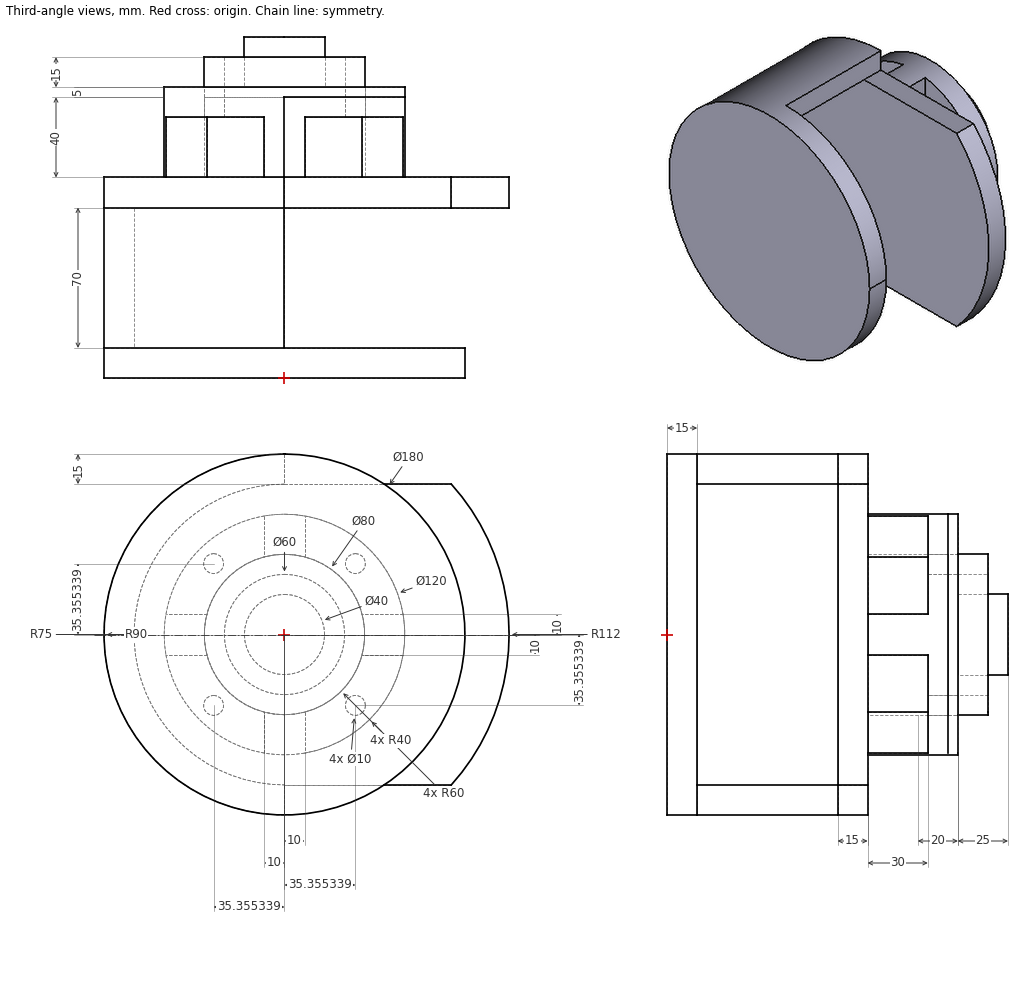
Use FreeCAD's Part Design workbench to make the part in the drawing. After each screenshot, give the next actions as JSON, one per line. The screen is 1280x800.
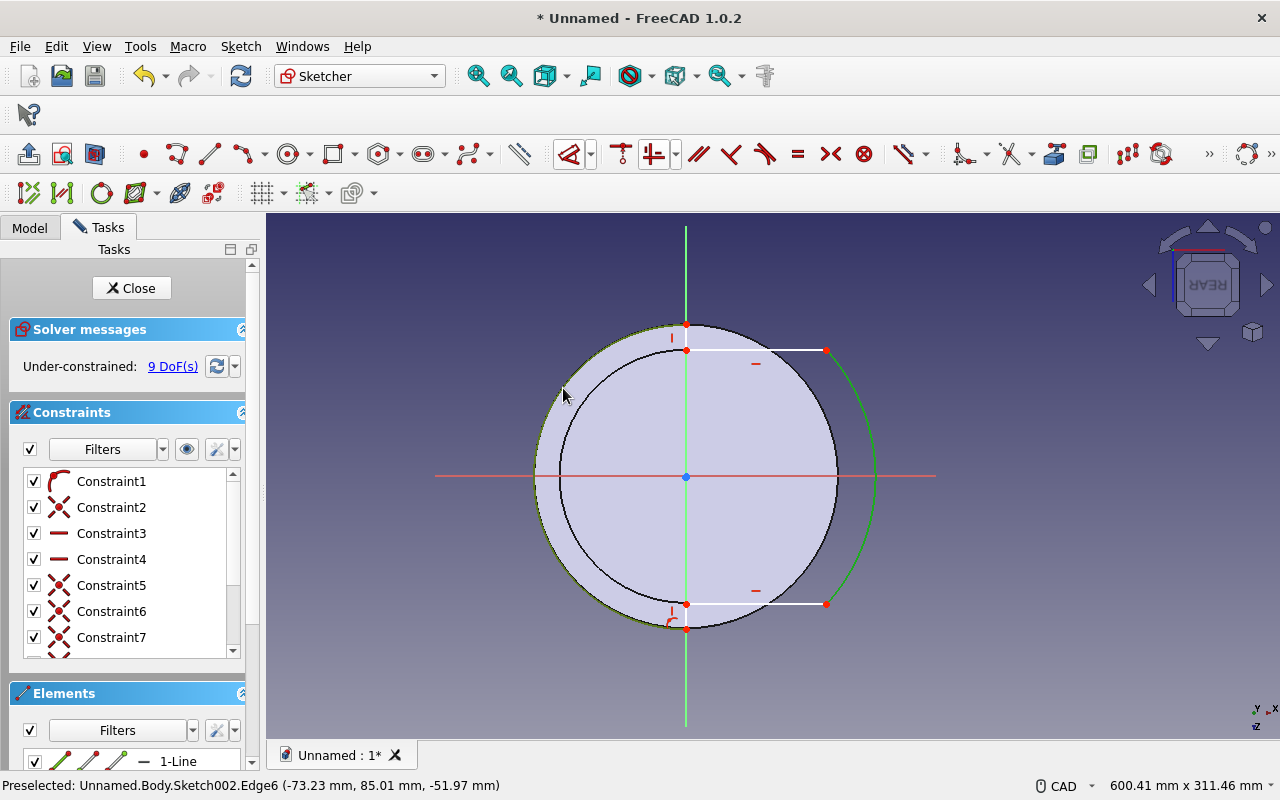
{"action": "left_click", "coordinate": [621, 154]}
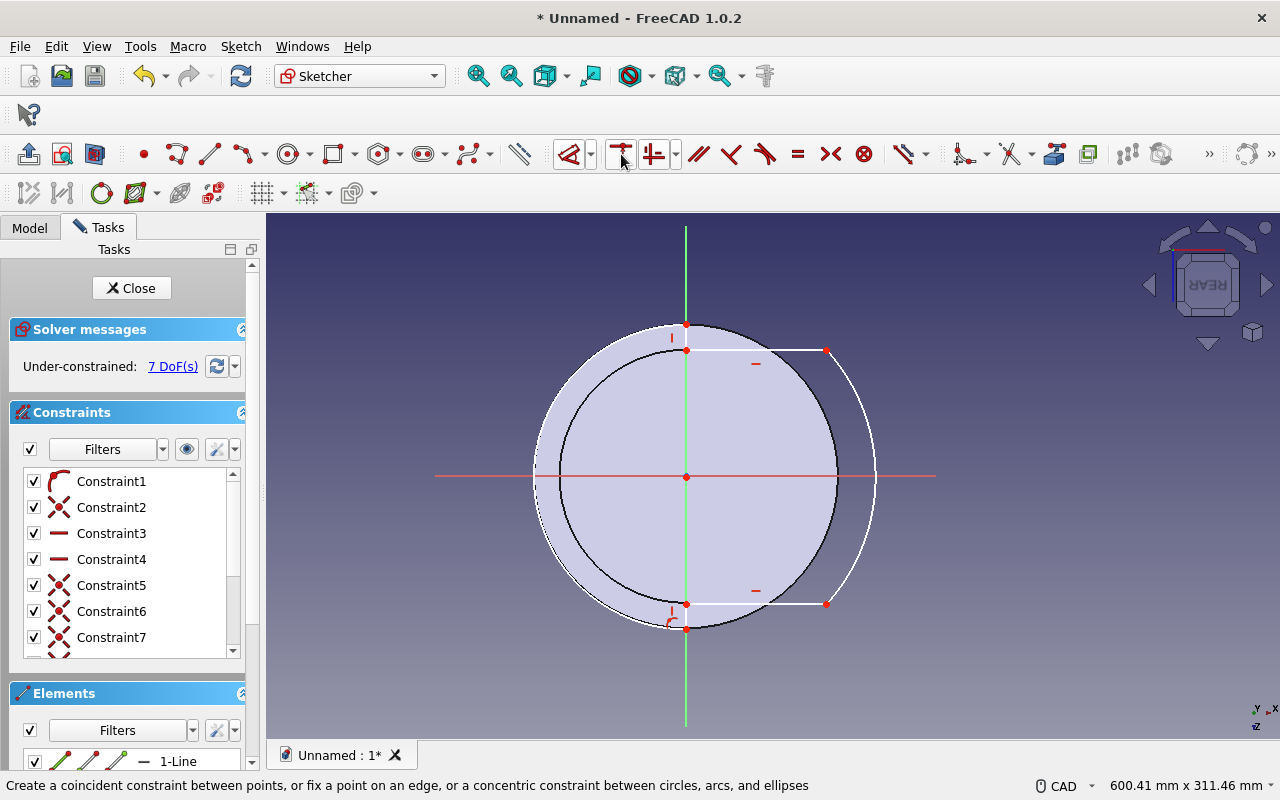
{"action": "left_click_drag", "start_coordinate": [676, 466], "coordinate": [696, 487]}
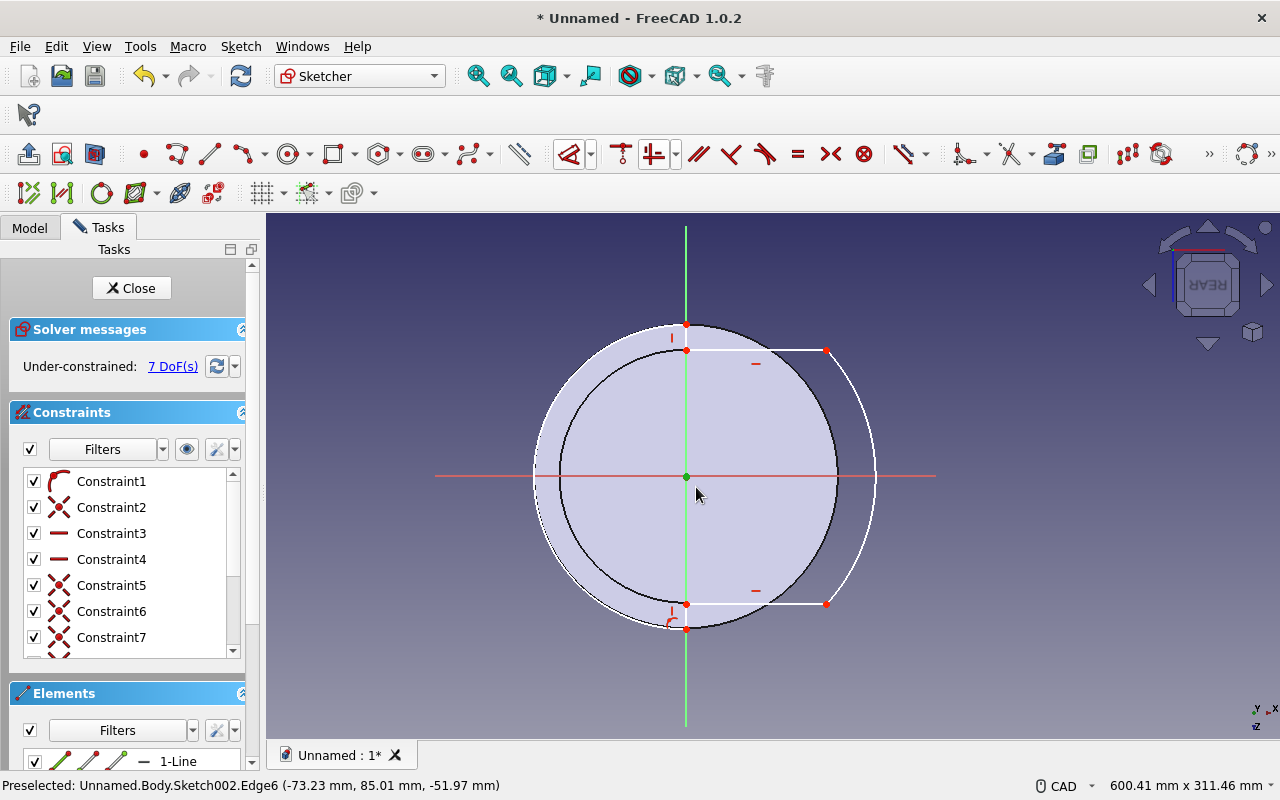
{"action": "left_click", "coordinate": [621, 154]}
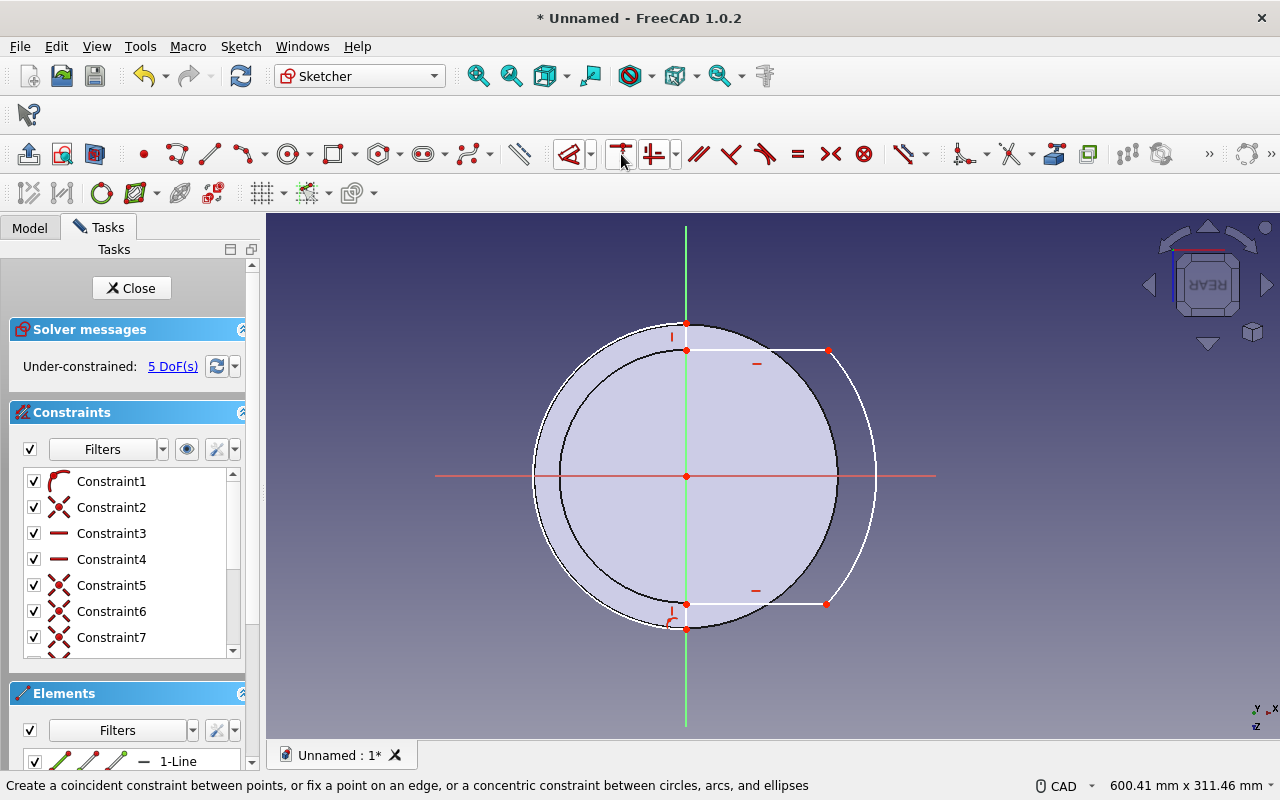
{"action": "left_click", "coordinate": [686, 604]}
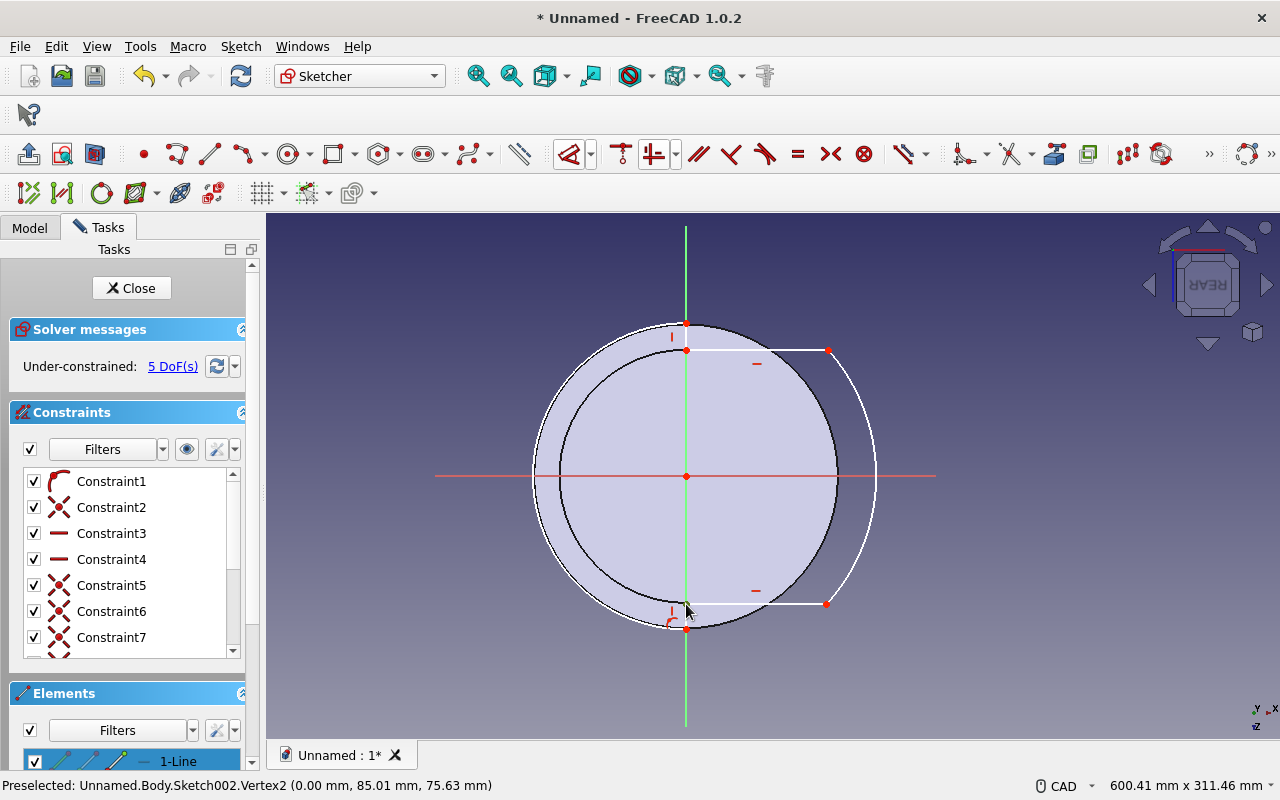
{"action": "left_click", "coordinate": [686, 350]}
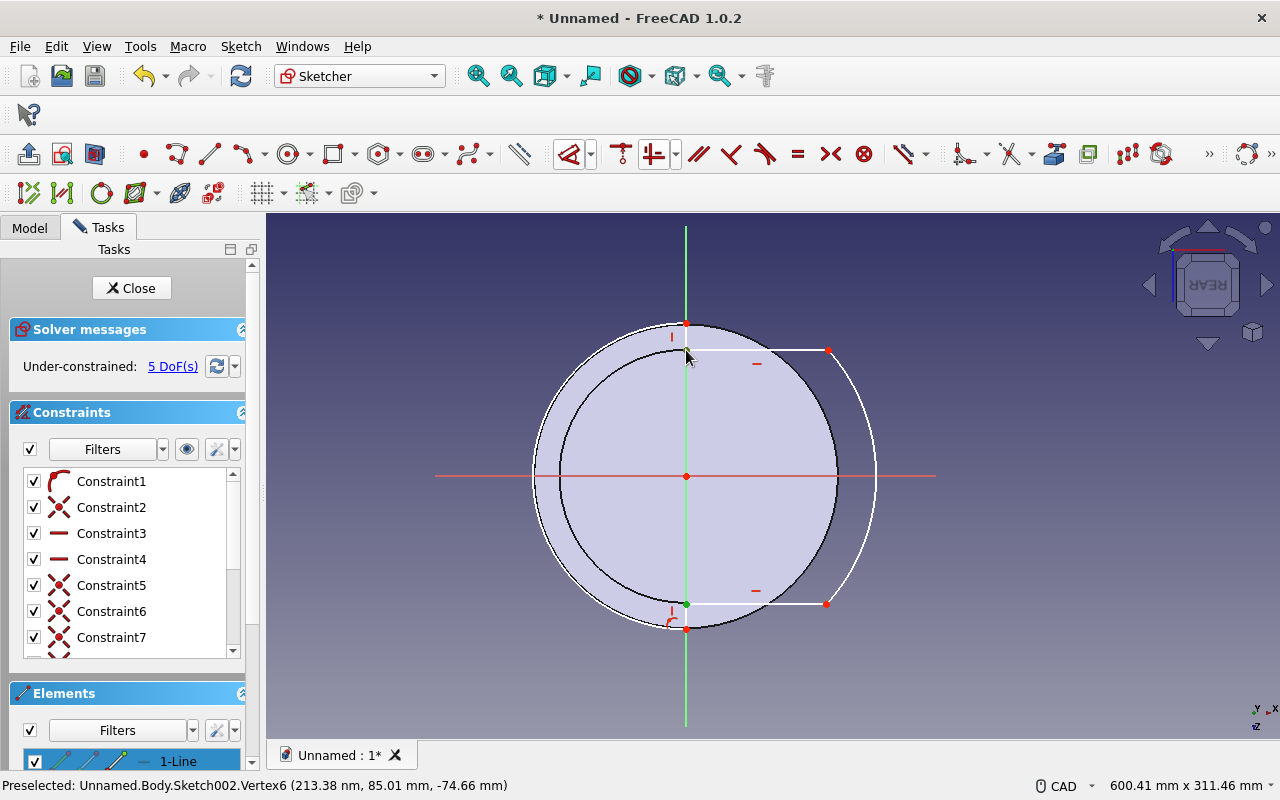
{"action": "left_click", "coordinate": [470, 476]}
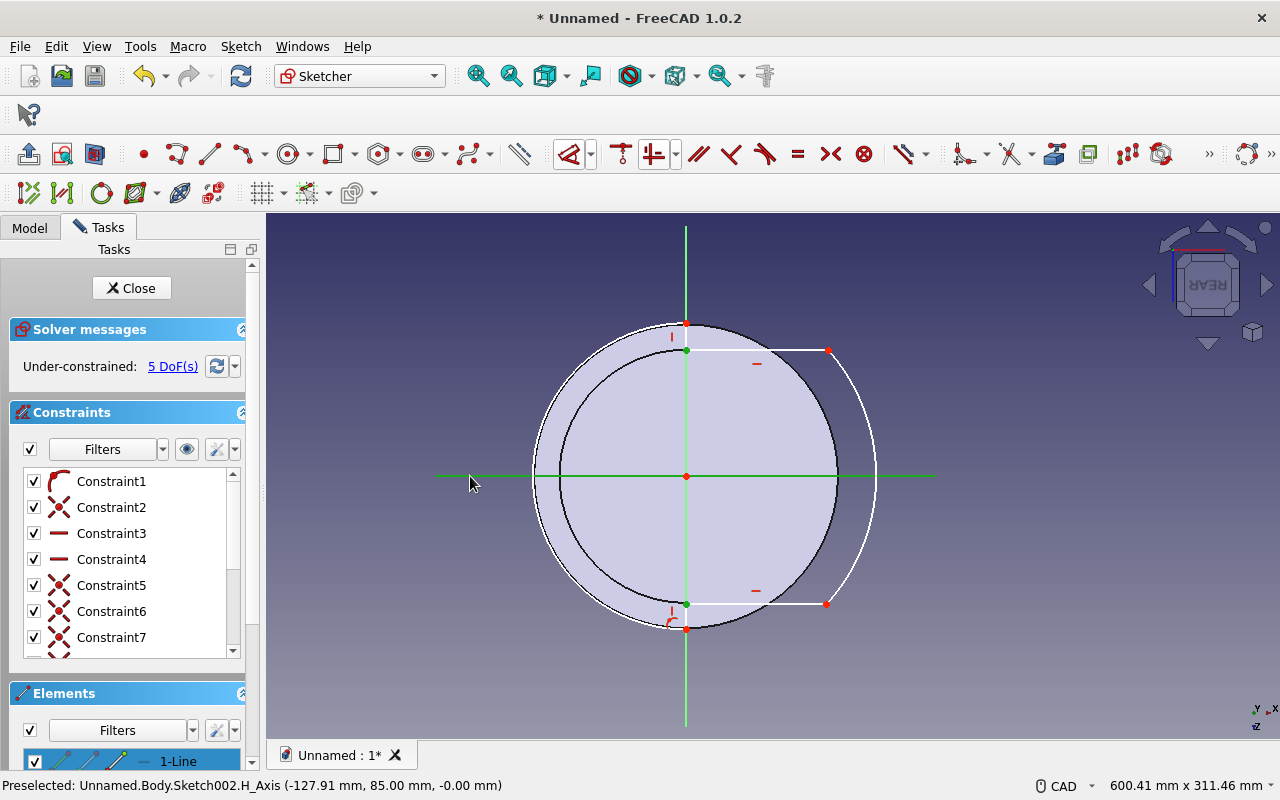
{"action": "left_click", "coordinate": [831, 154]}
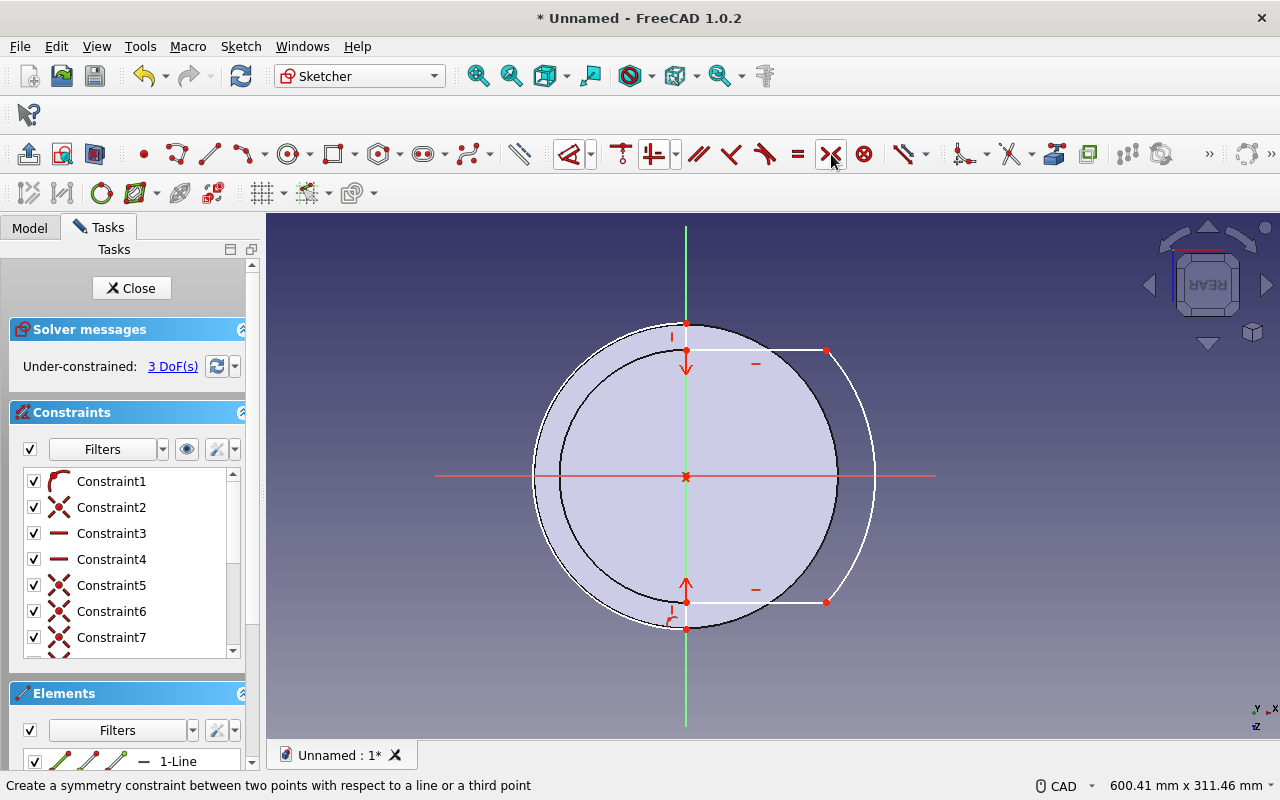
{"action": "left_click", "coordinate": [867, 531]}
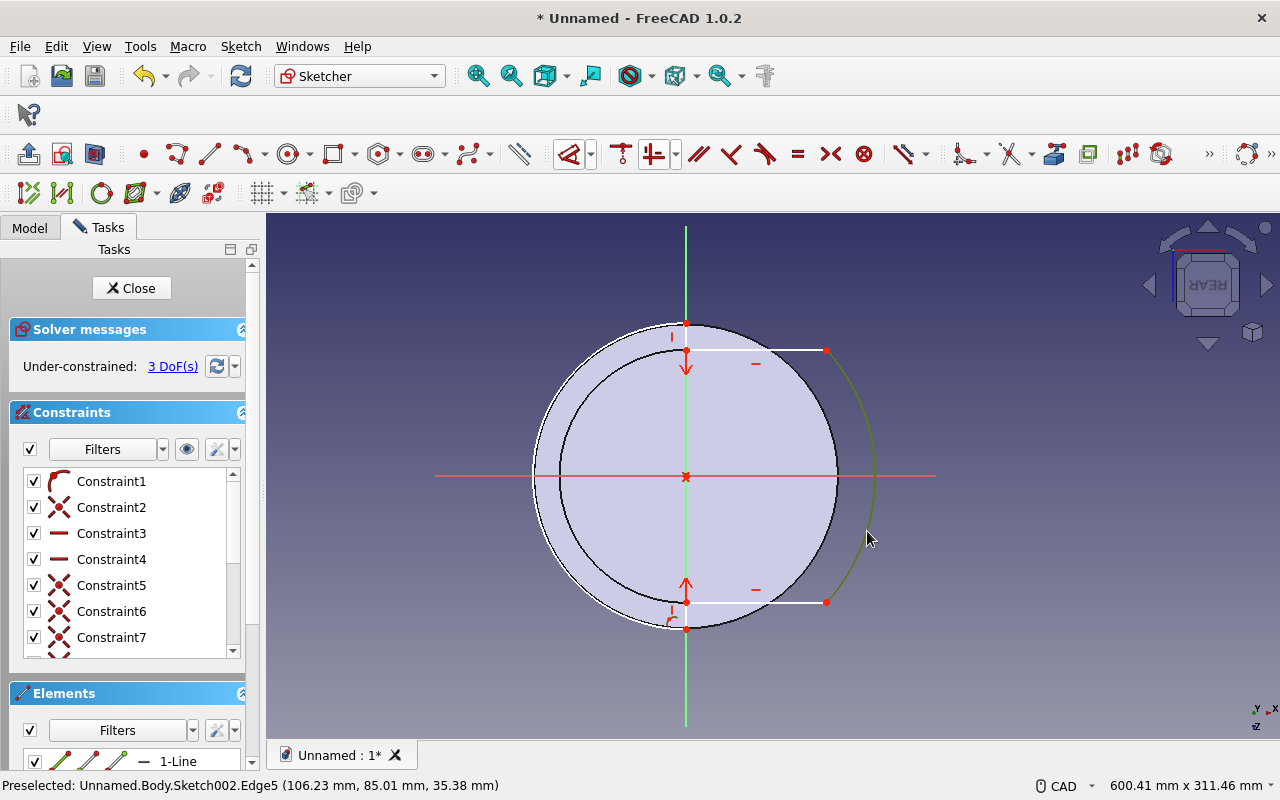
{"action": "left_click", "coordinate": [590, 154]}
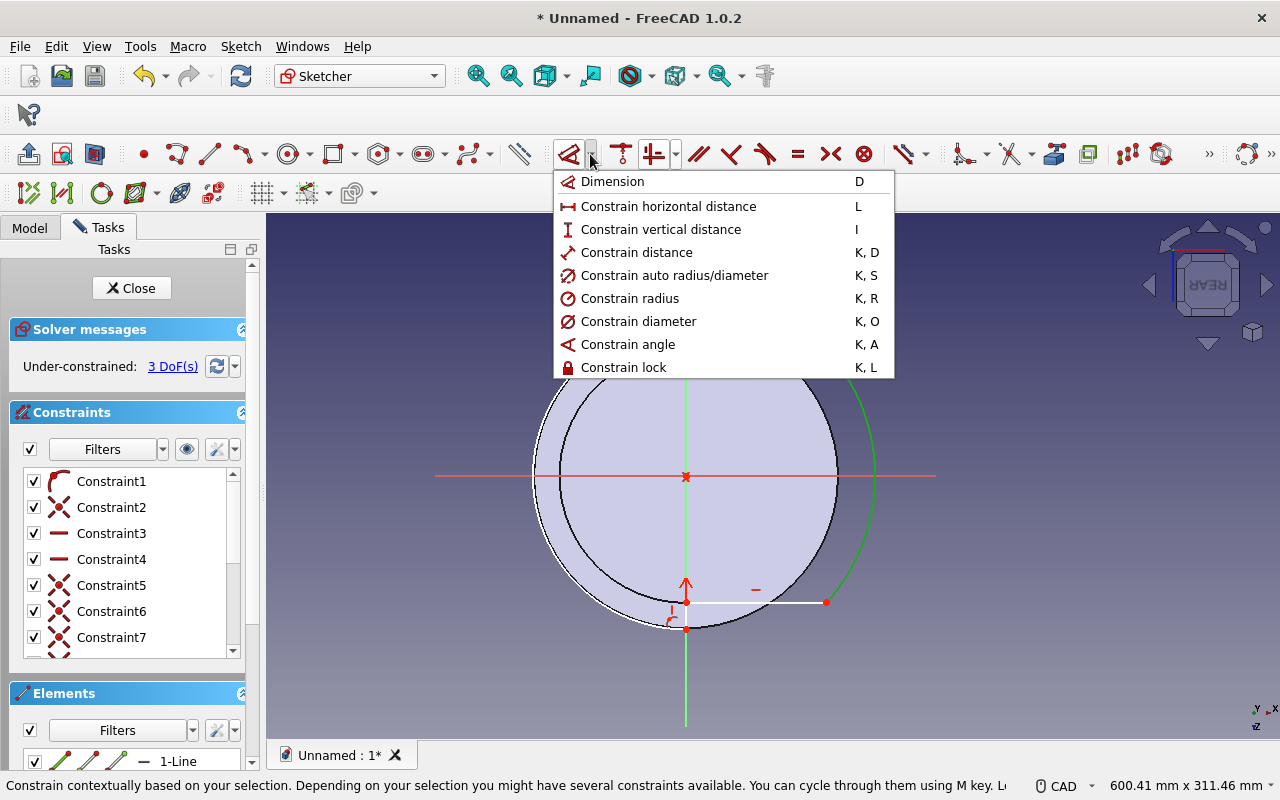
{"action": "left_click", "coordinate": [724, 298]}